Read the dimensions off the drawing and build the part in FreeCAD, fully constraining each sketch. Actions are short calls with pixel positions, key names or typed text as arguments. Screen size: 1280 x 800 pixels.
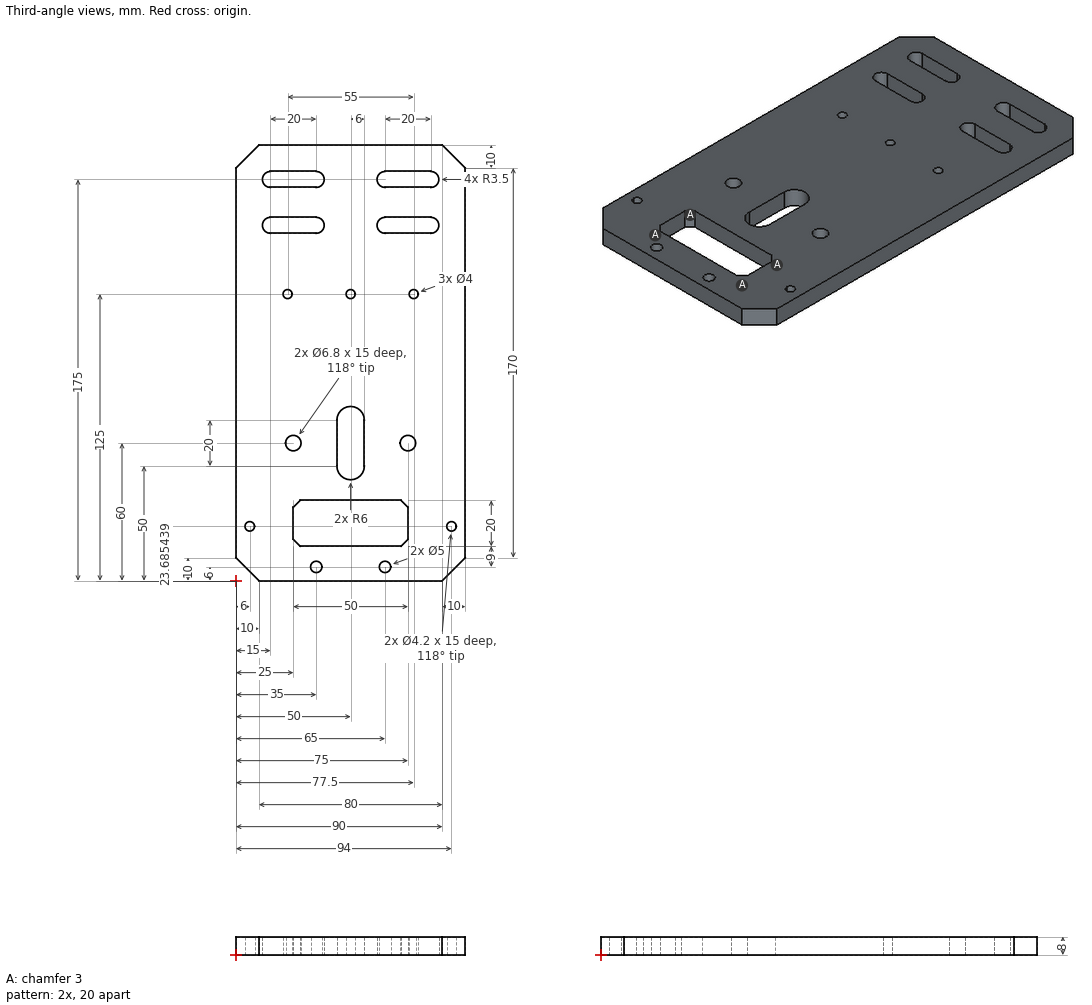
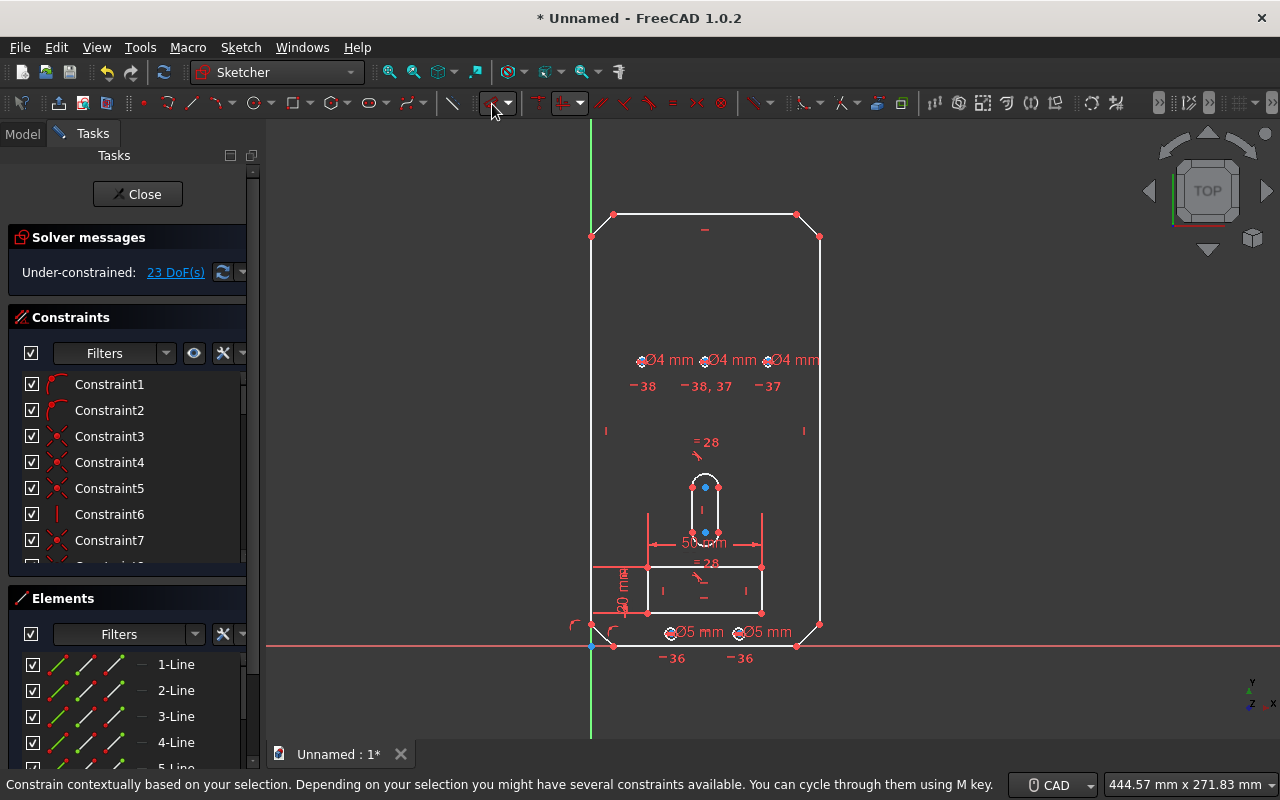
scroll(698, 543, up, 6)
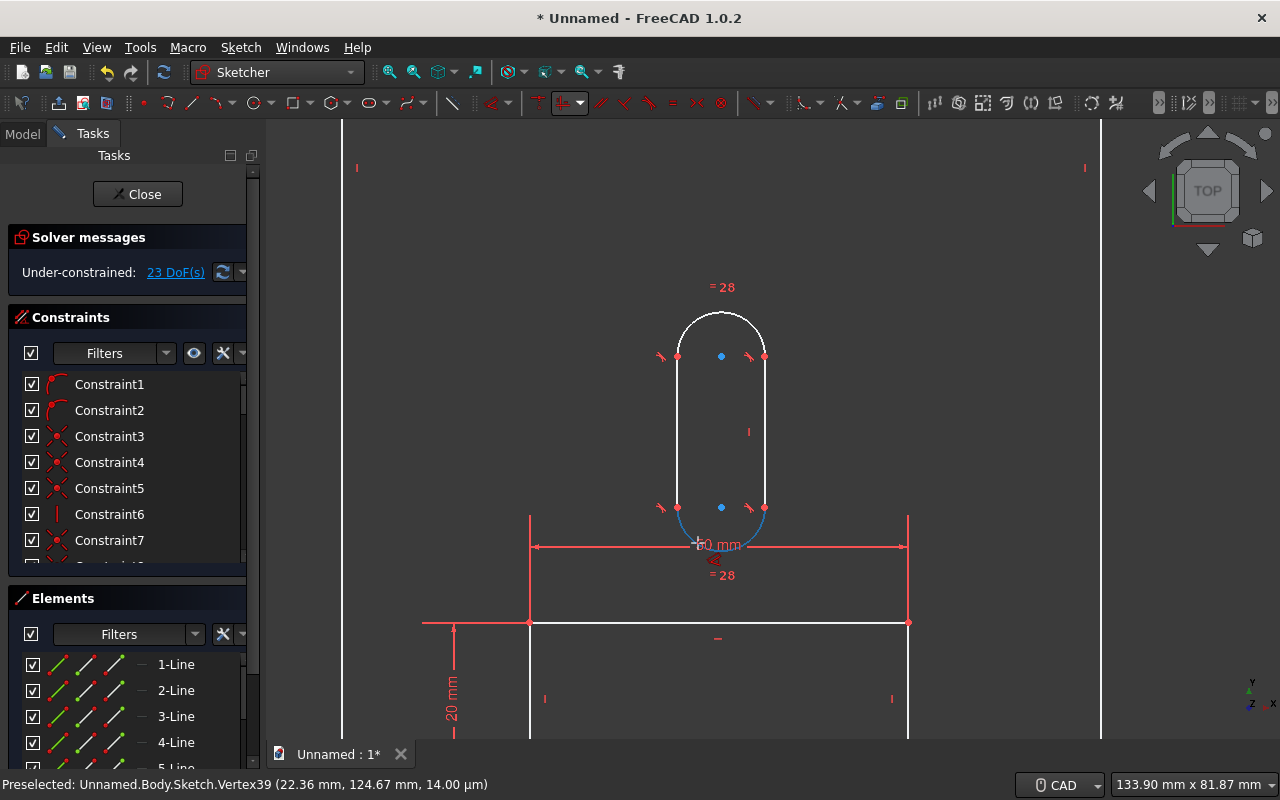
click(696, 543)
click(678, 569)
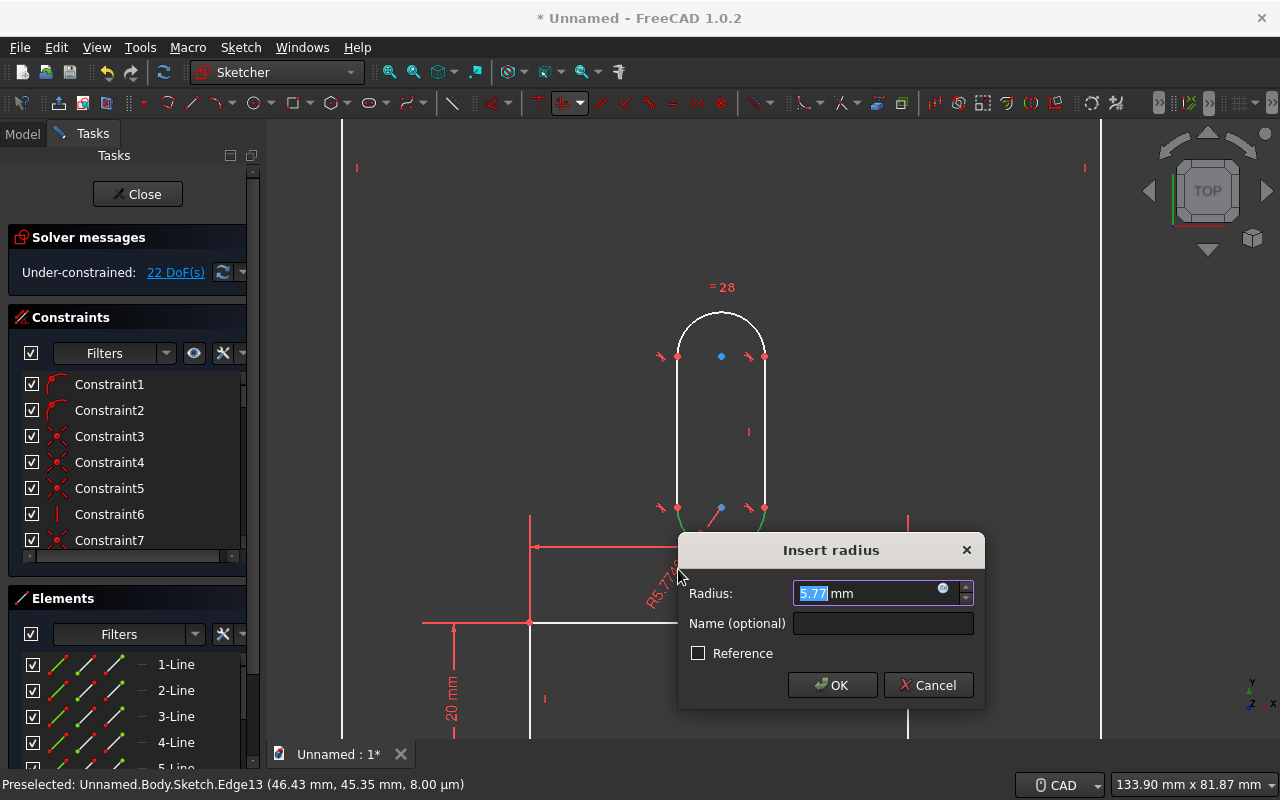
text(6)
key(Return)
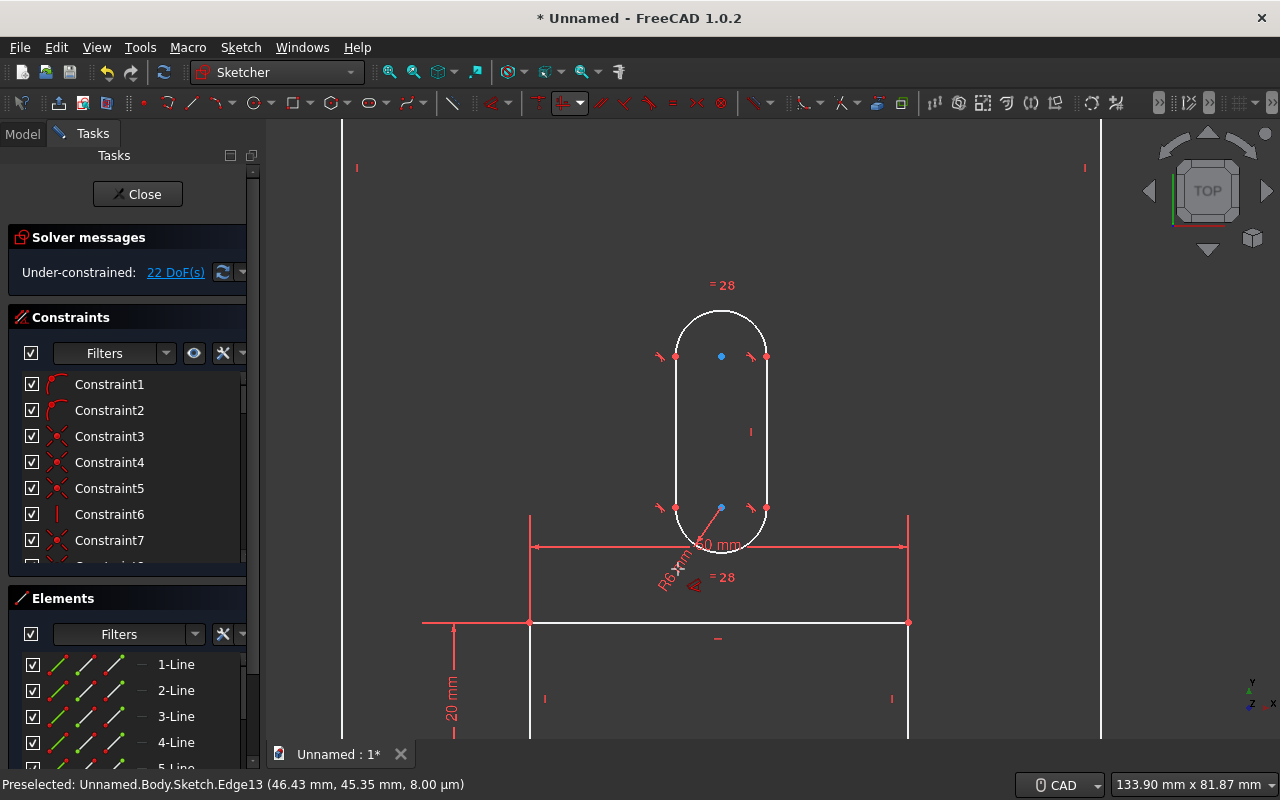
scroll(698, 543, down, 6)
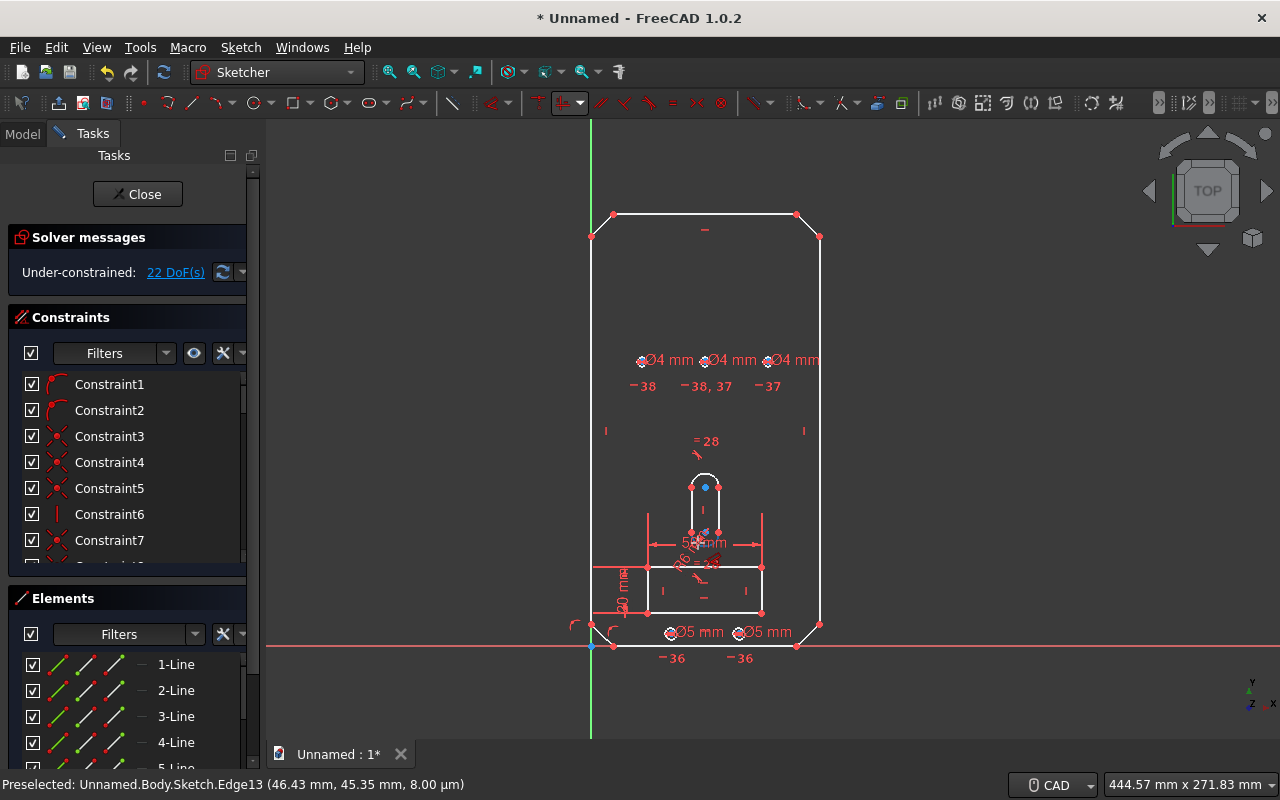
scroll(739, 634, up, 6)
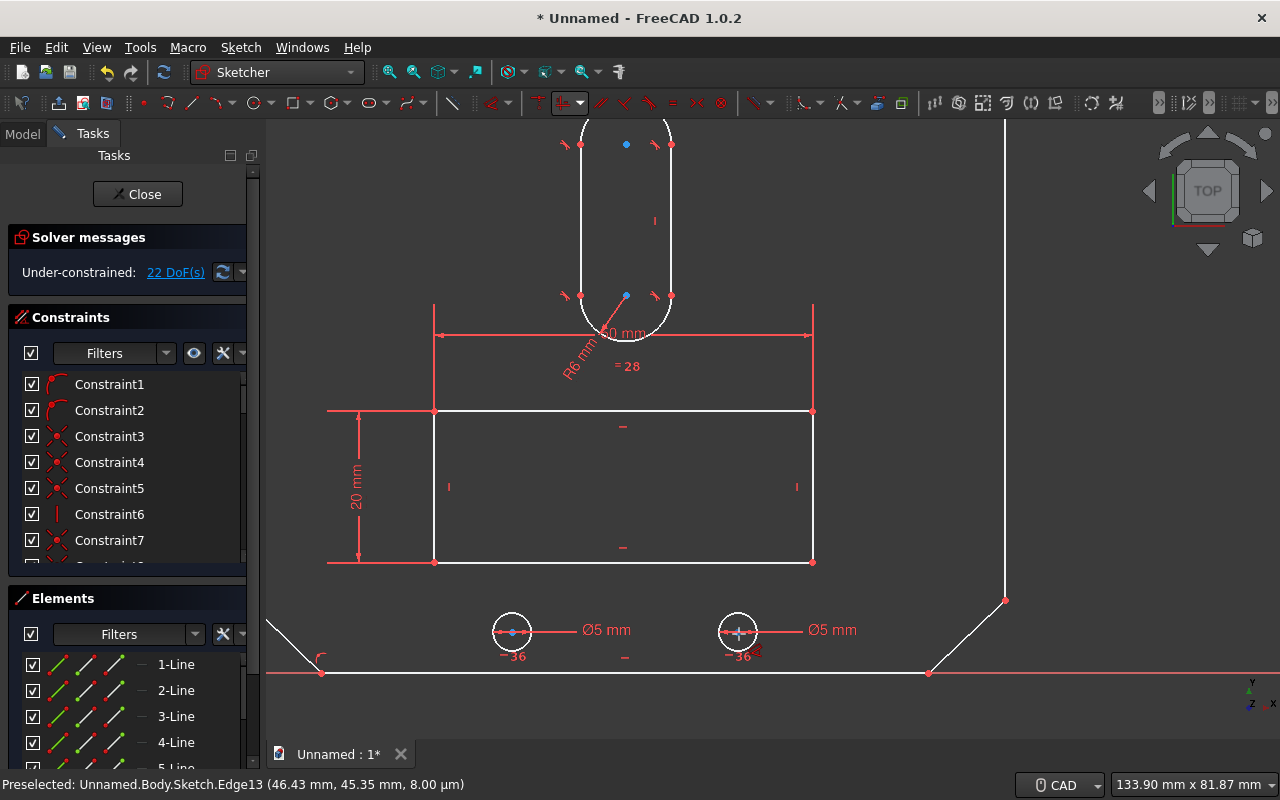
click(738, 632)
click(772, 653)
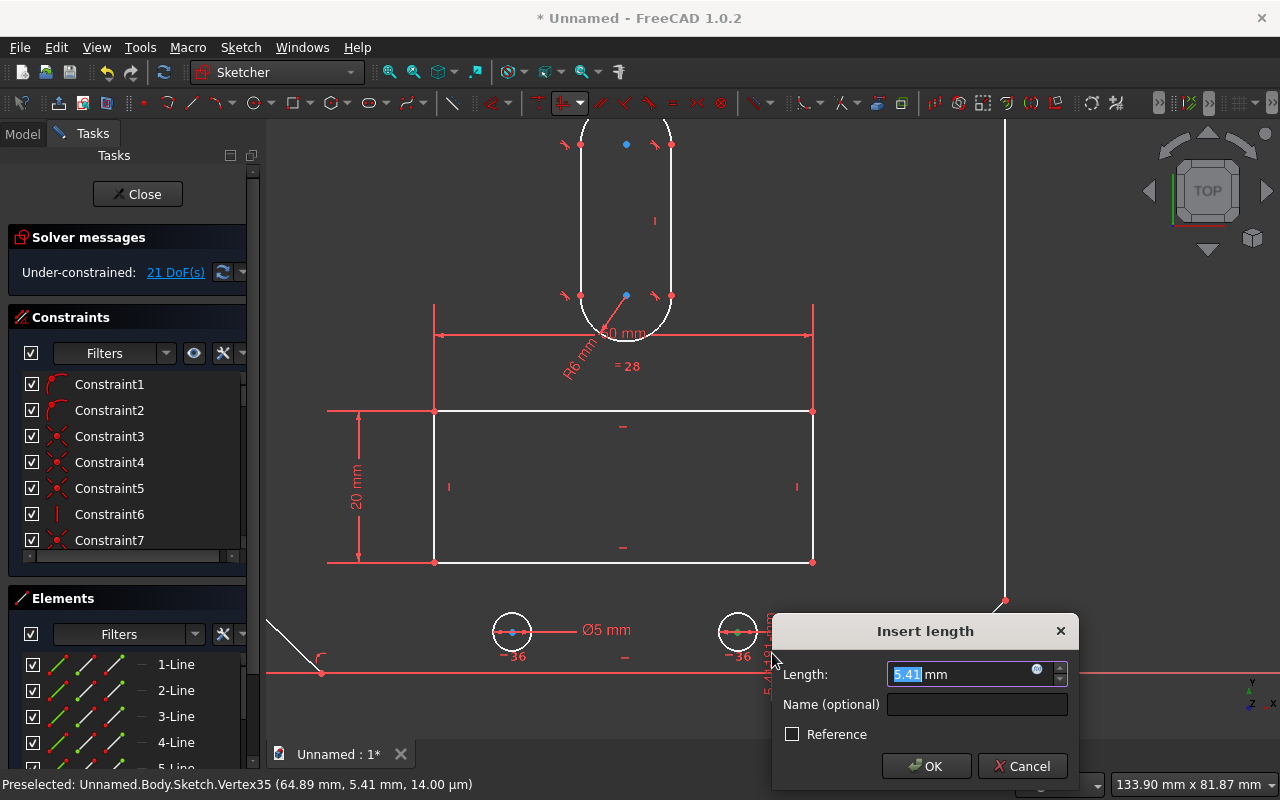
text(6)
key(Return)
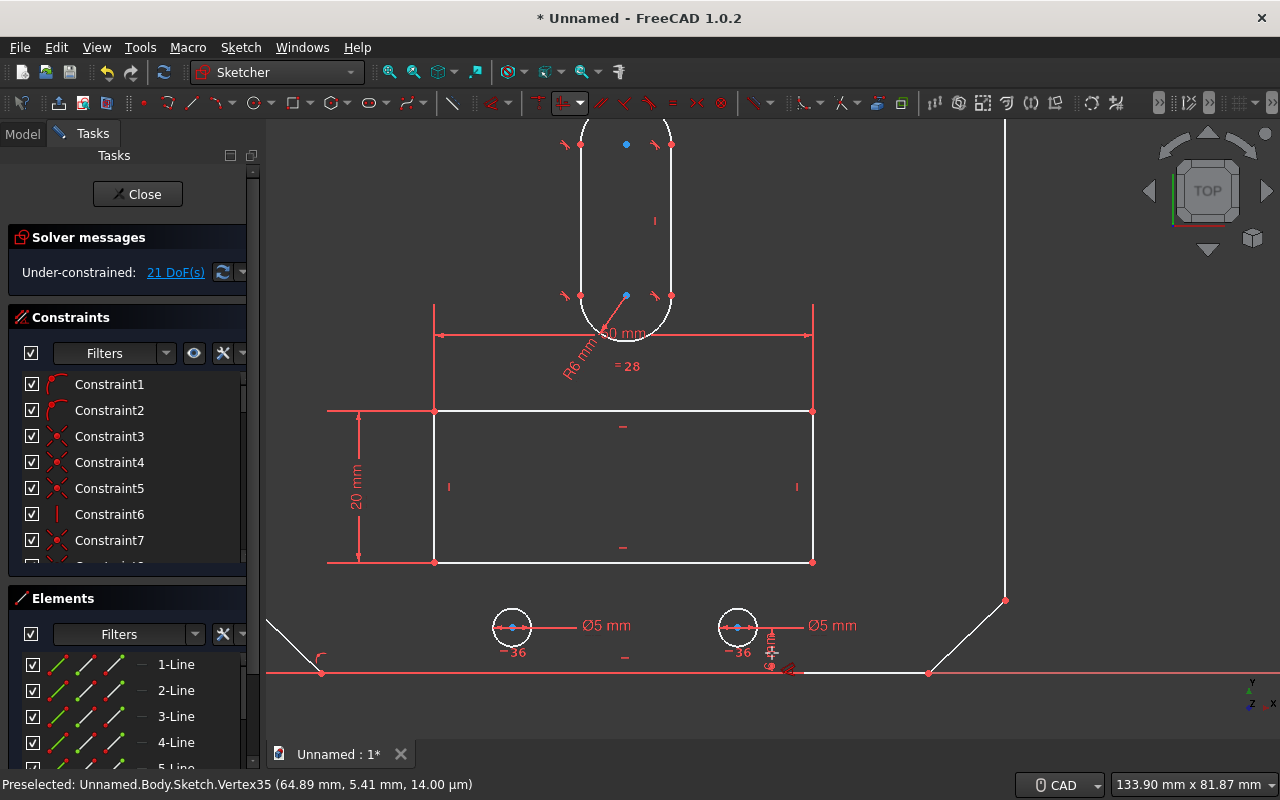
click(504, 673)
click(625, 707)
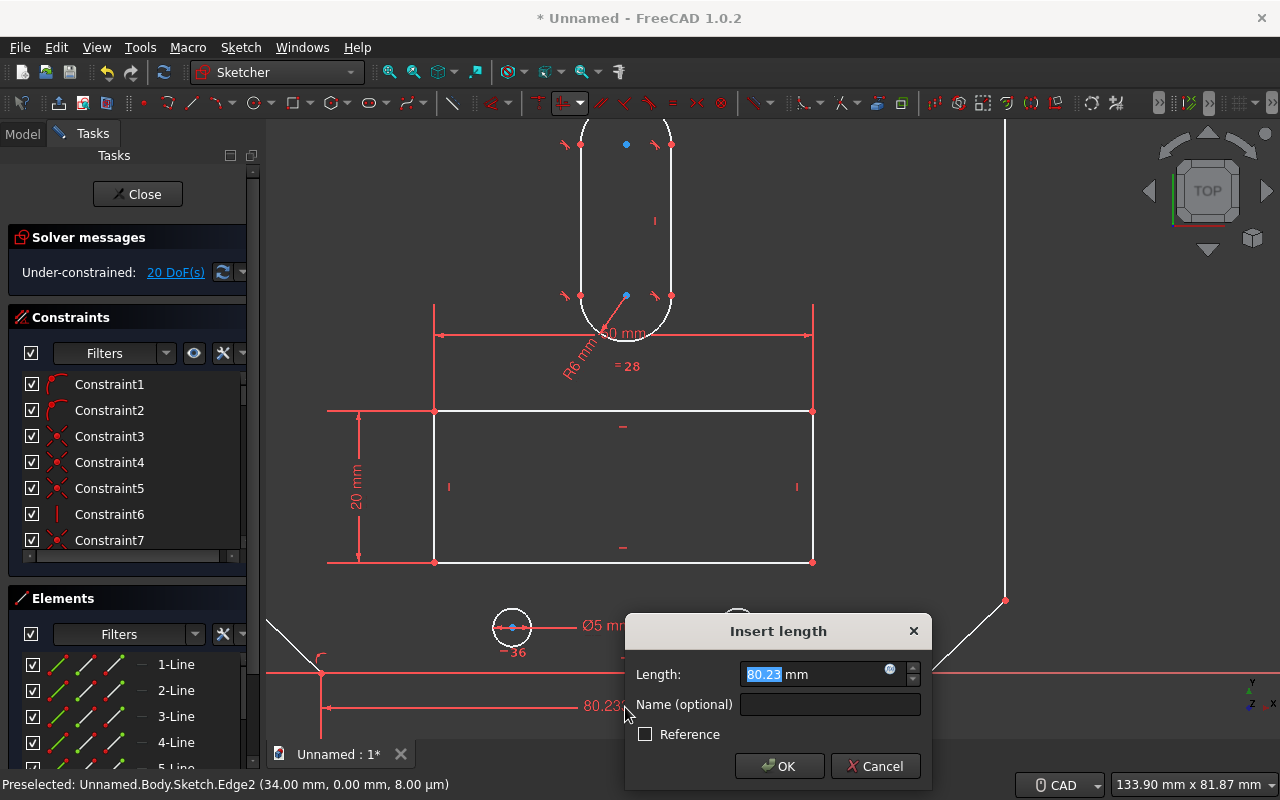
text(80)
key(Return)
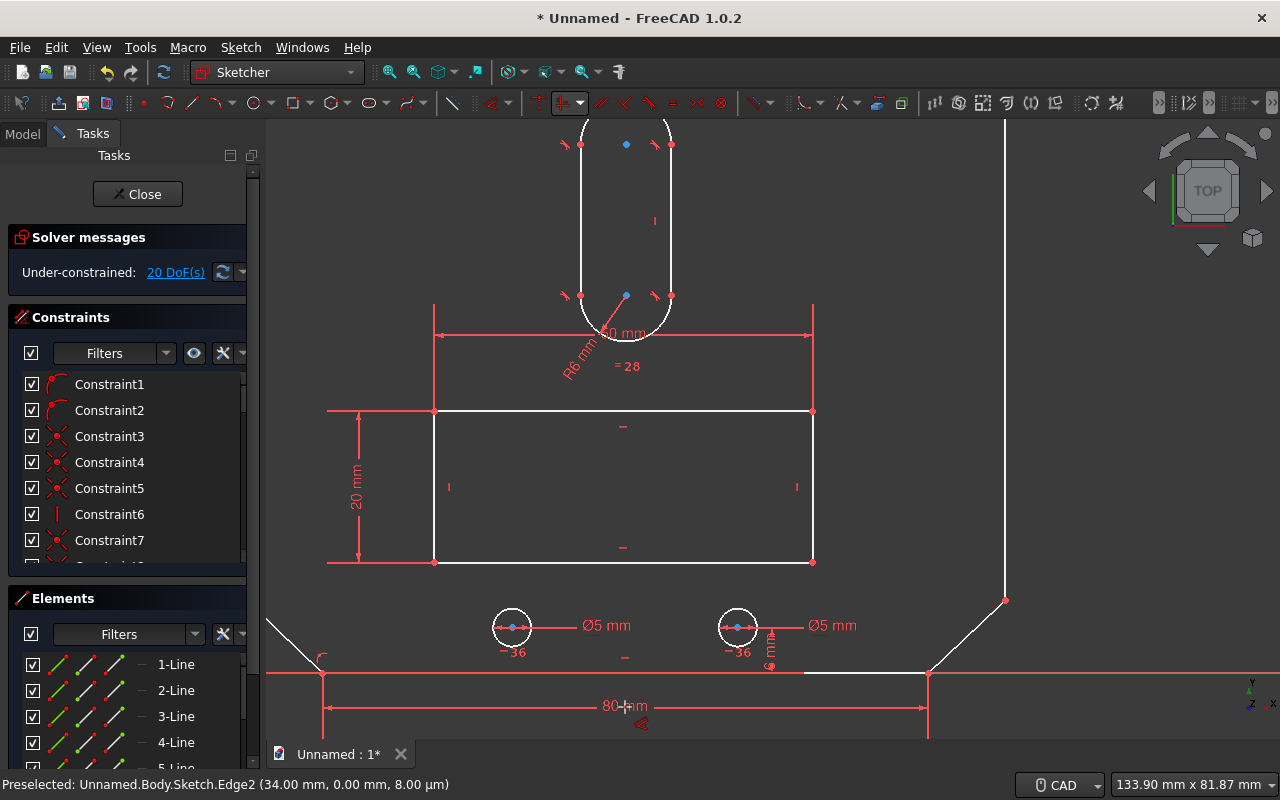
scroll(739, 634, down, 6)